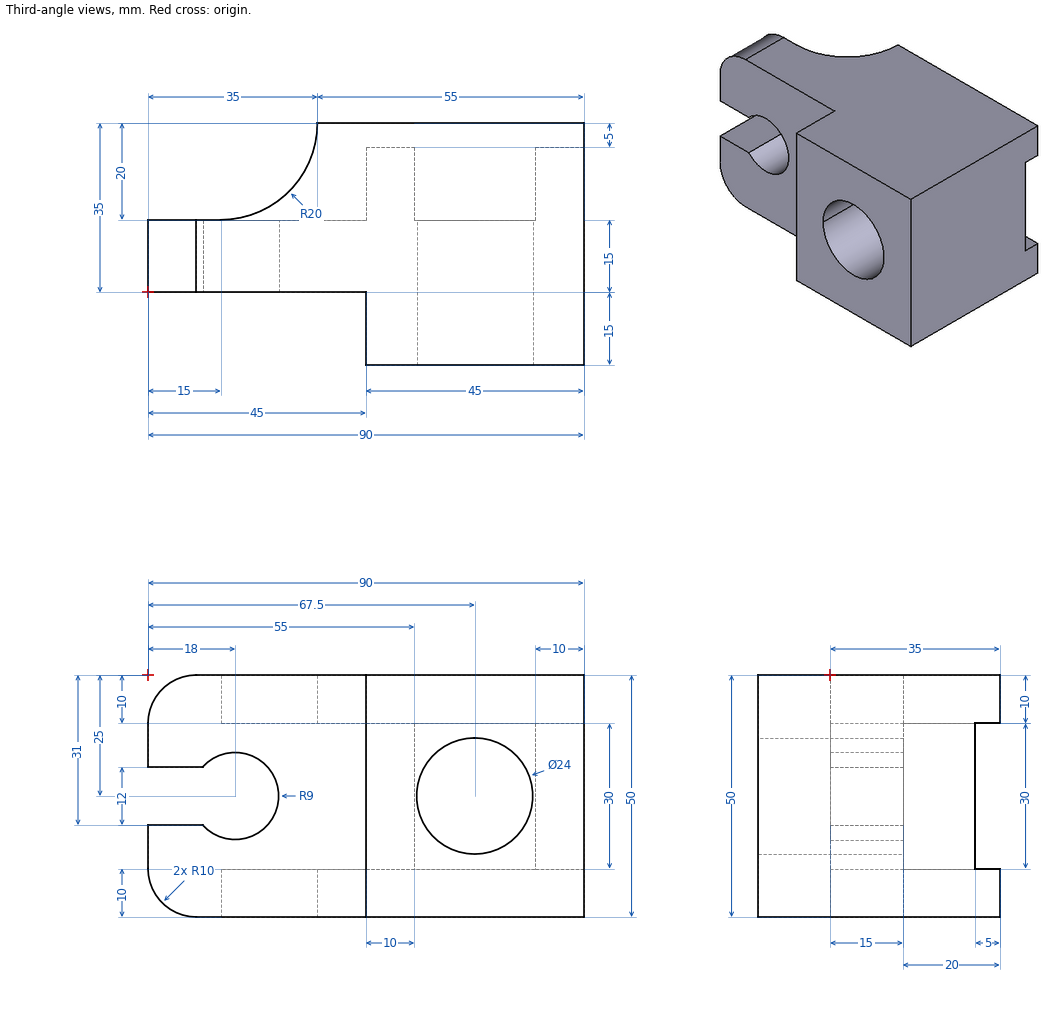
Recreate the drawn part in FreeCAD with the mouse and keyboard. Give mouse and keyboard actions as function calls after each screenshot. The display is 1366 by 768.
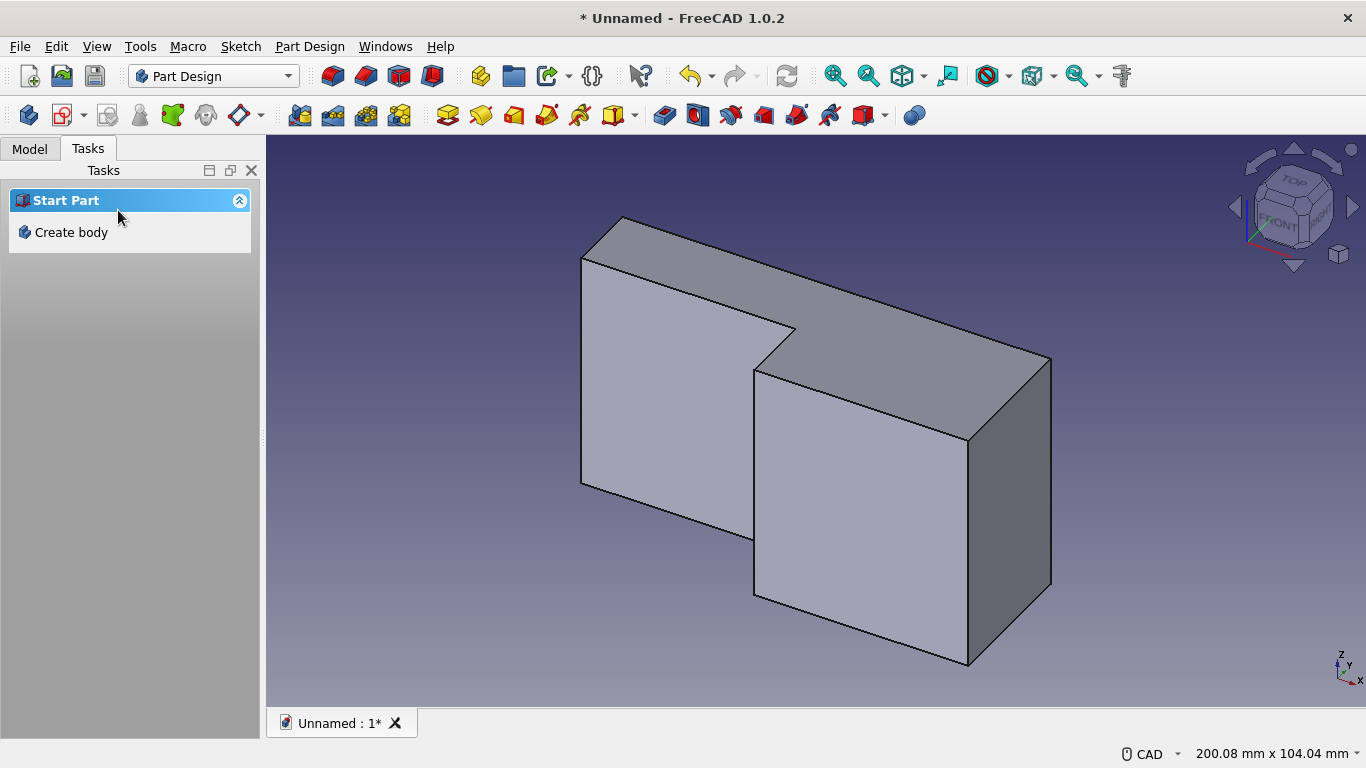
click(918, 368)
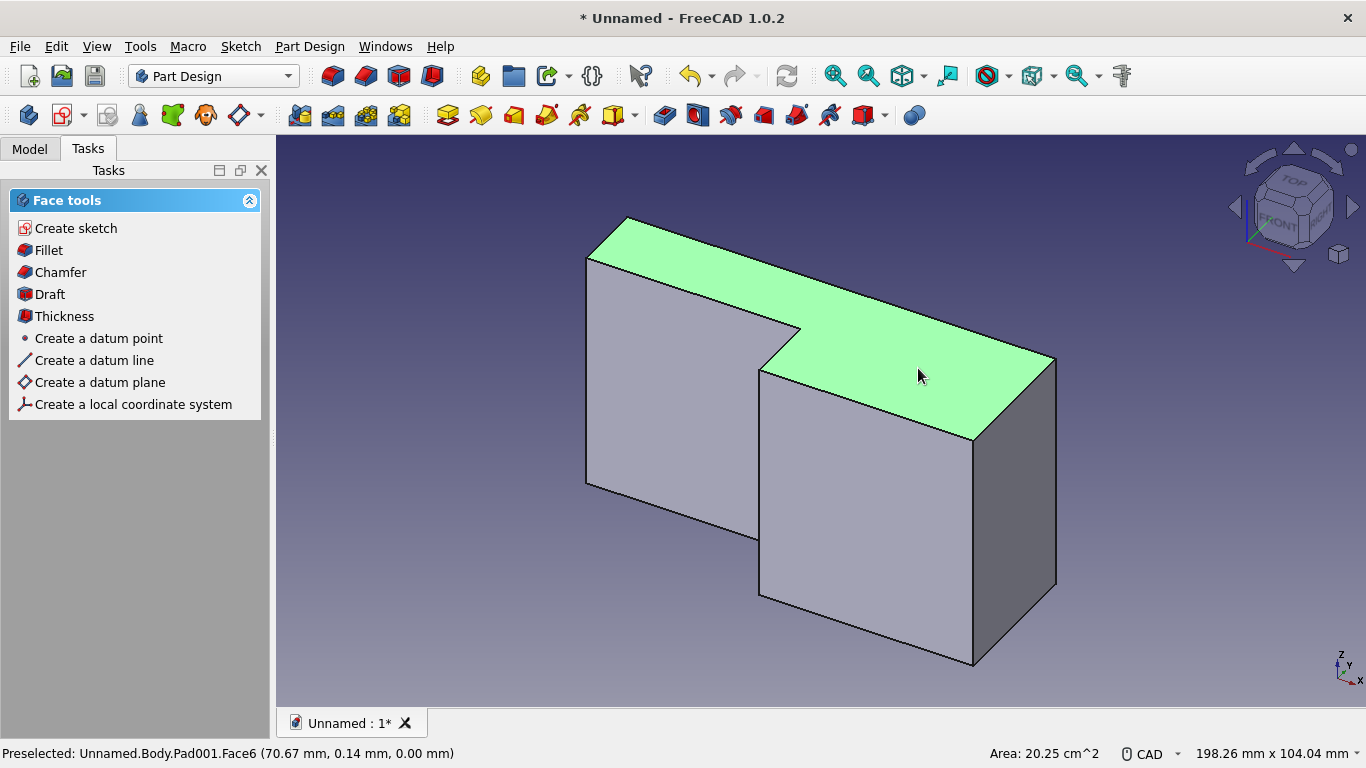
click(62, 116)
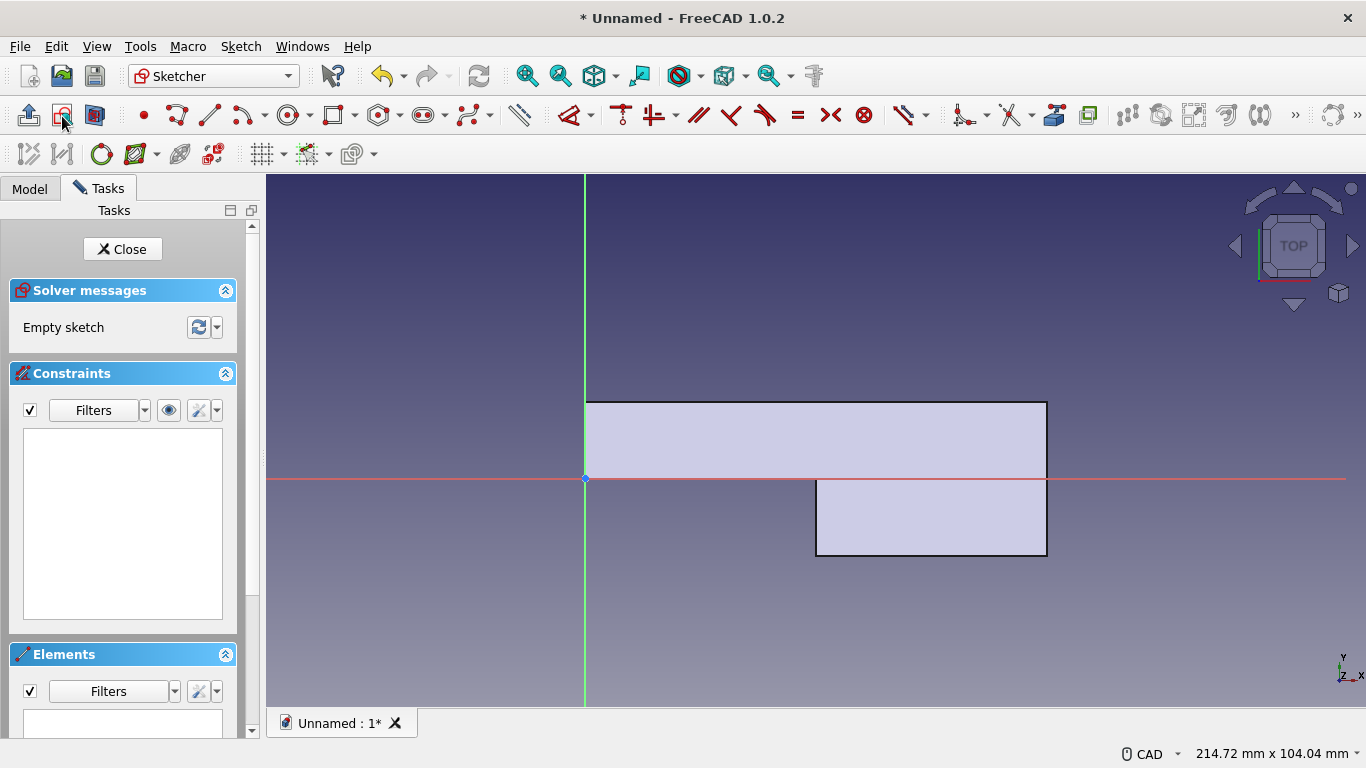
scroll(955, 285, up, 2)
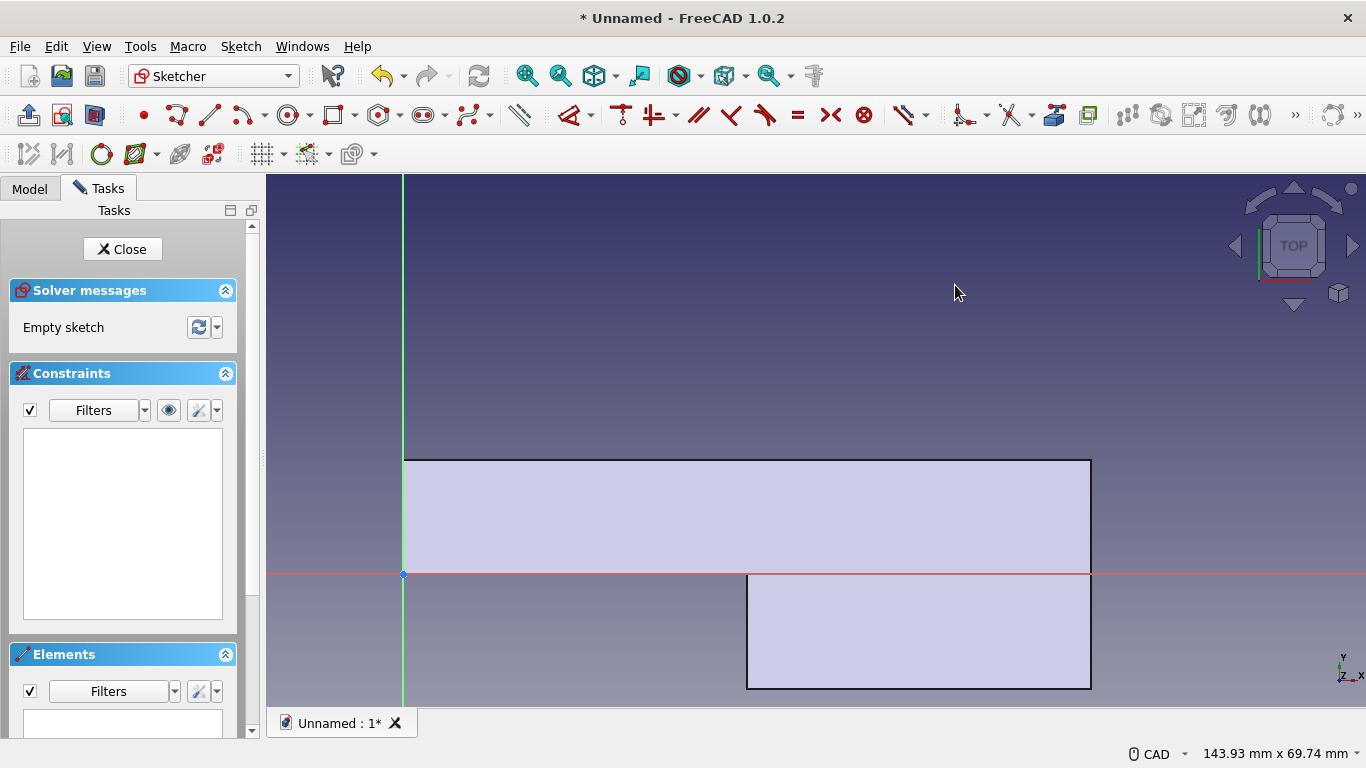
click(332, 116)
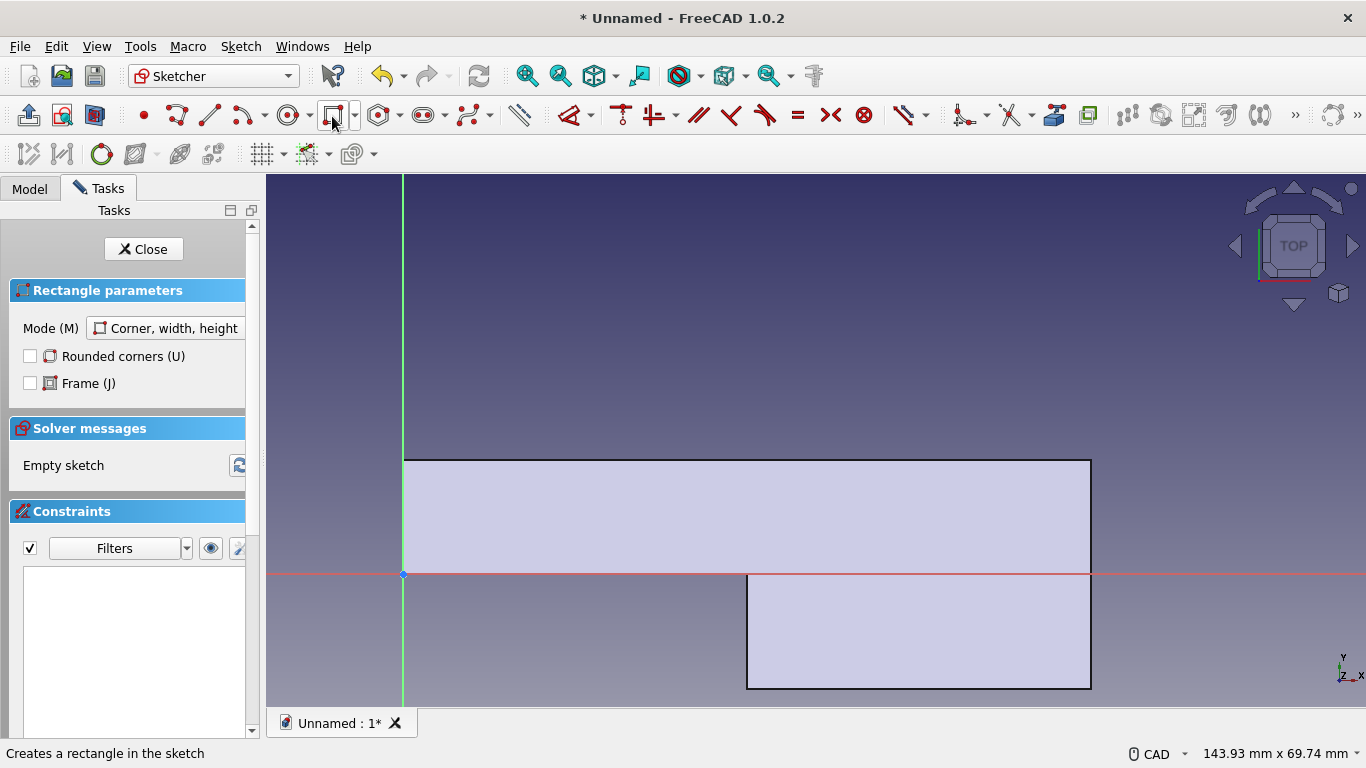
click(671, 307)
click(1091, 460)
key(Escape)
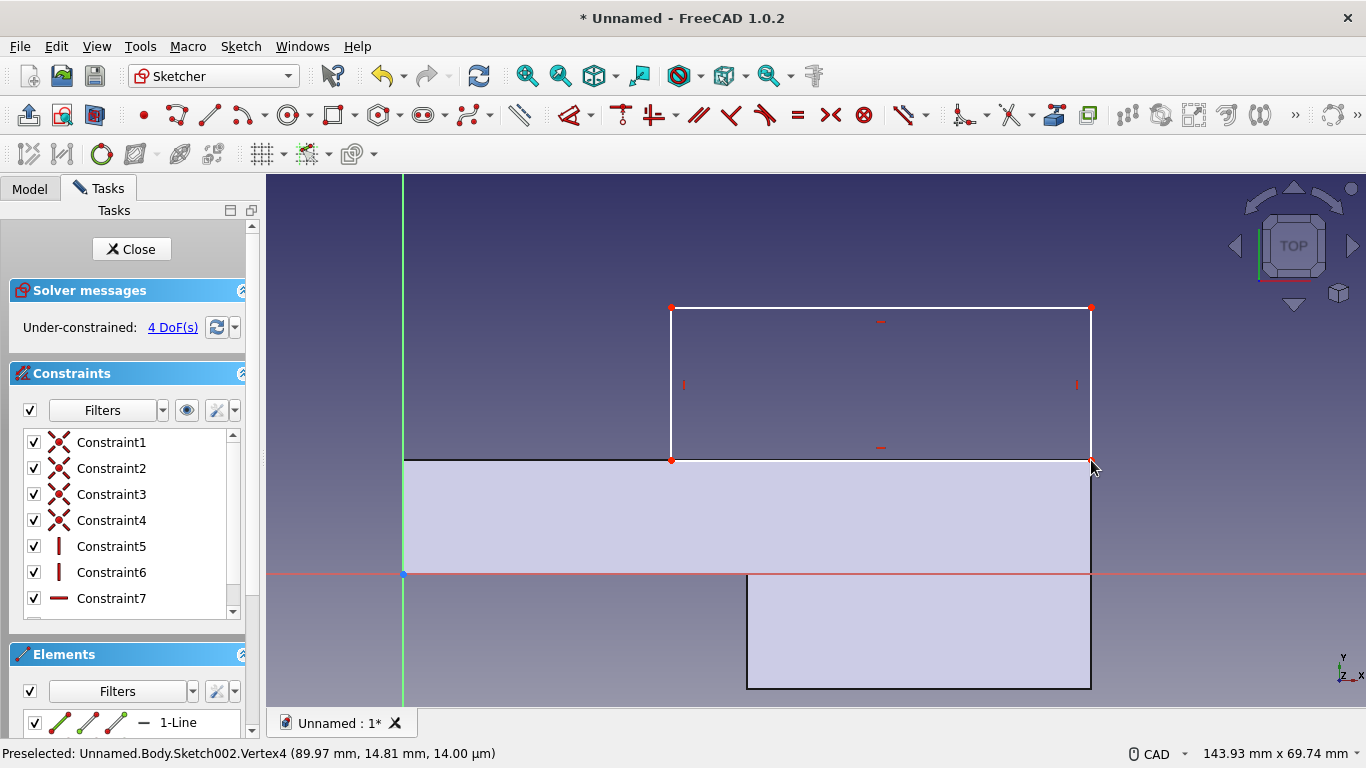
click(568, 116)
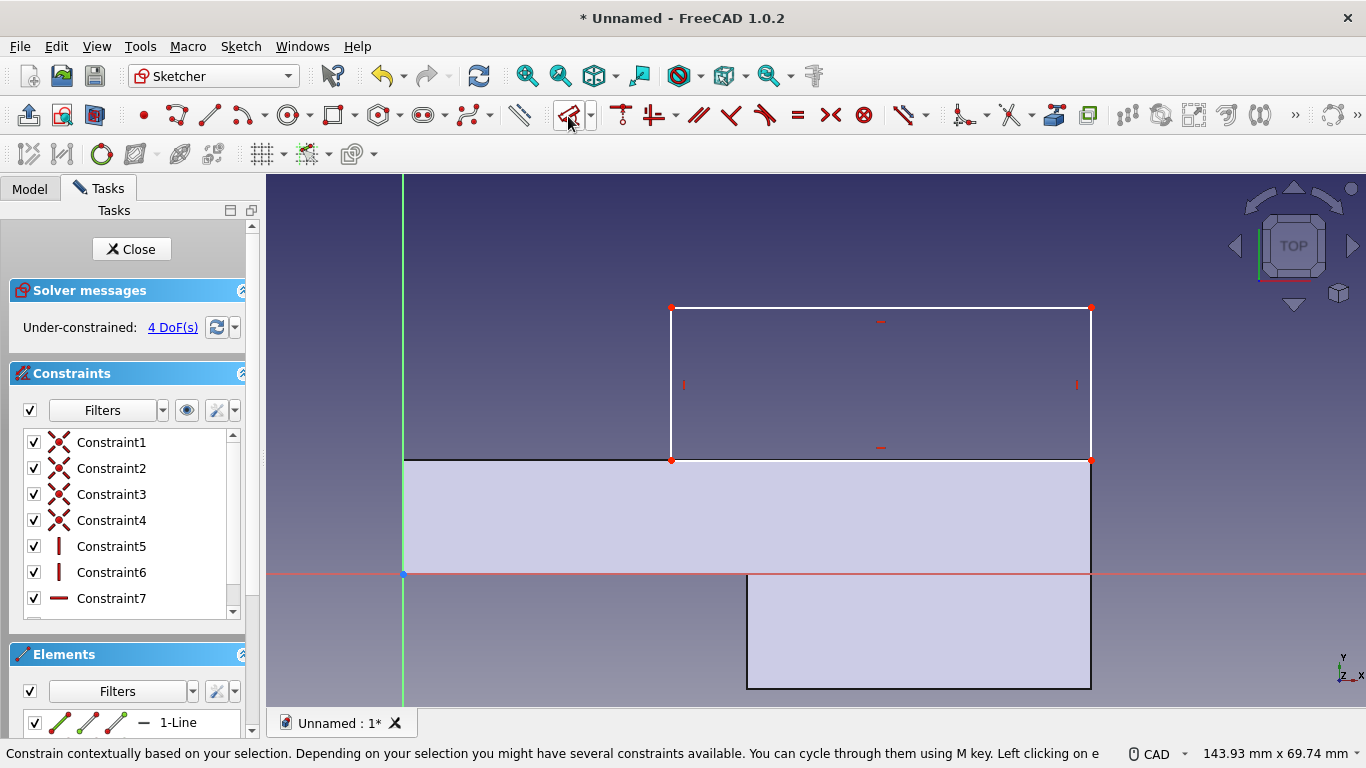
click(671, 354)
click(637, 385)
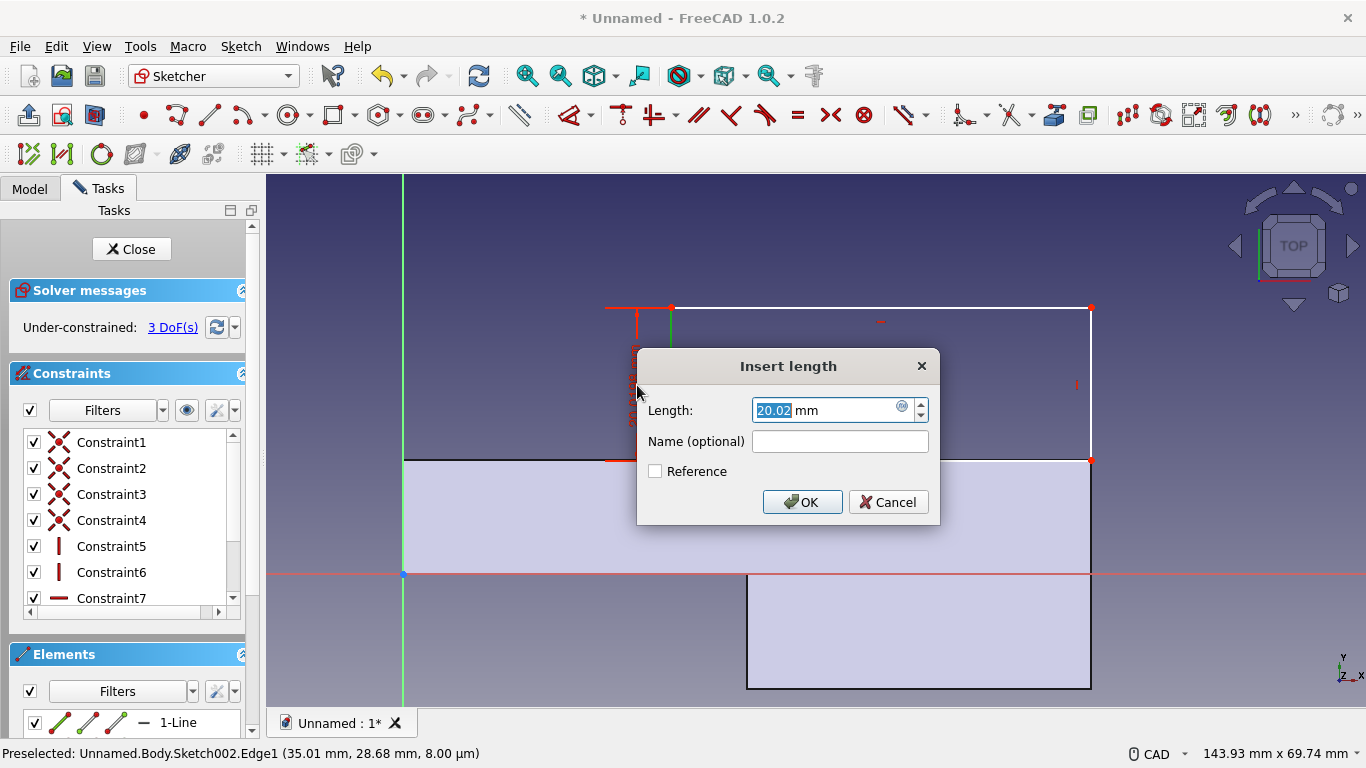
text(20)
key(Return)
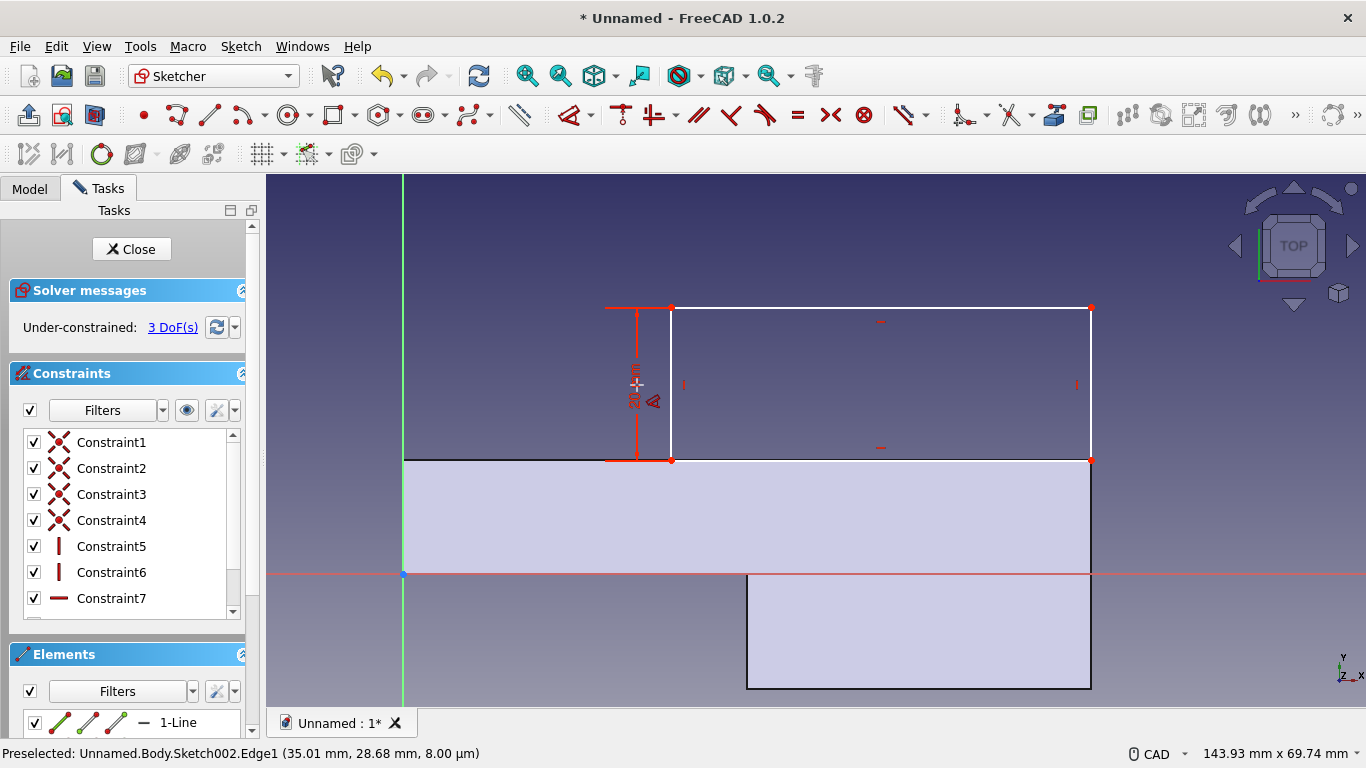
click(797, 461)
click(881, 495)